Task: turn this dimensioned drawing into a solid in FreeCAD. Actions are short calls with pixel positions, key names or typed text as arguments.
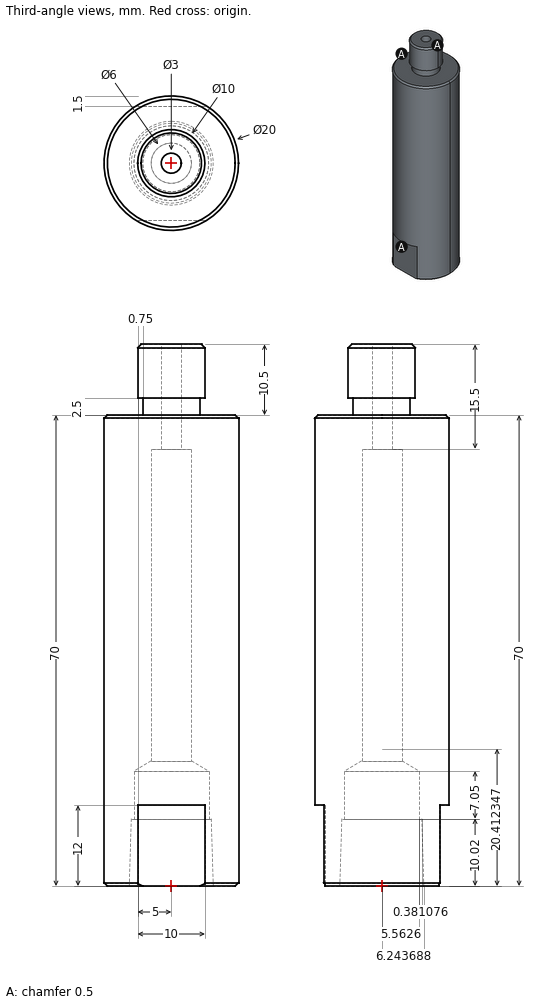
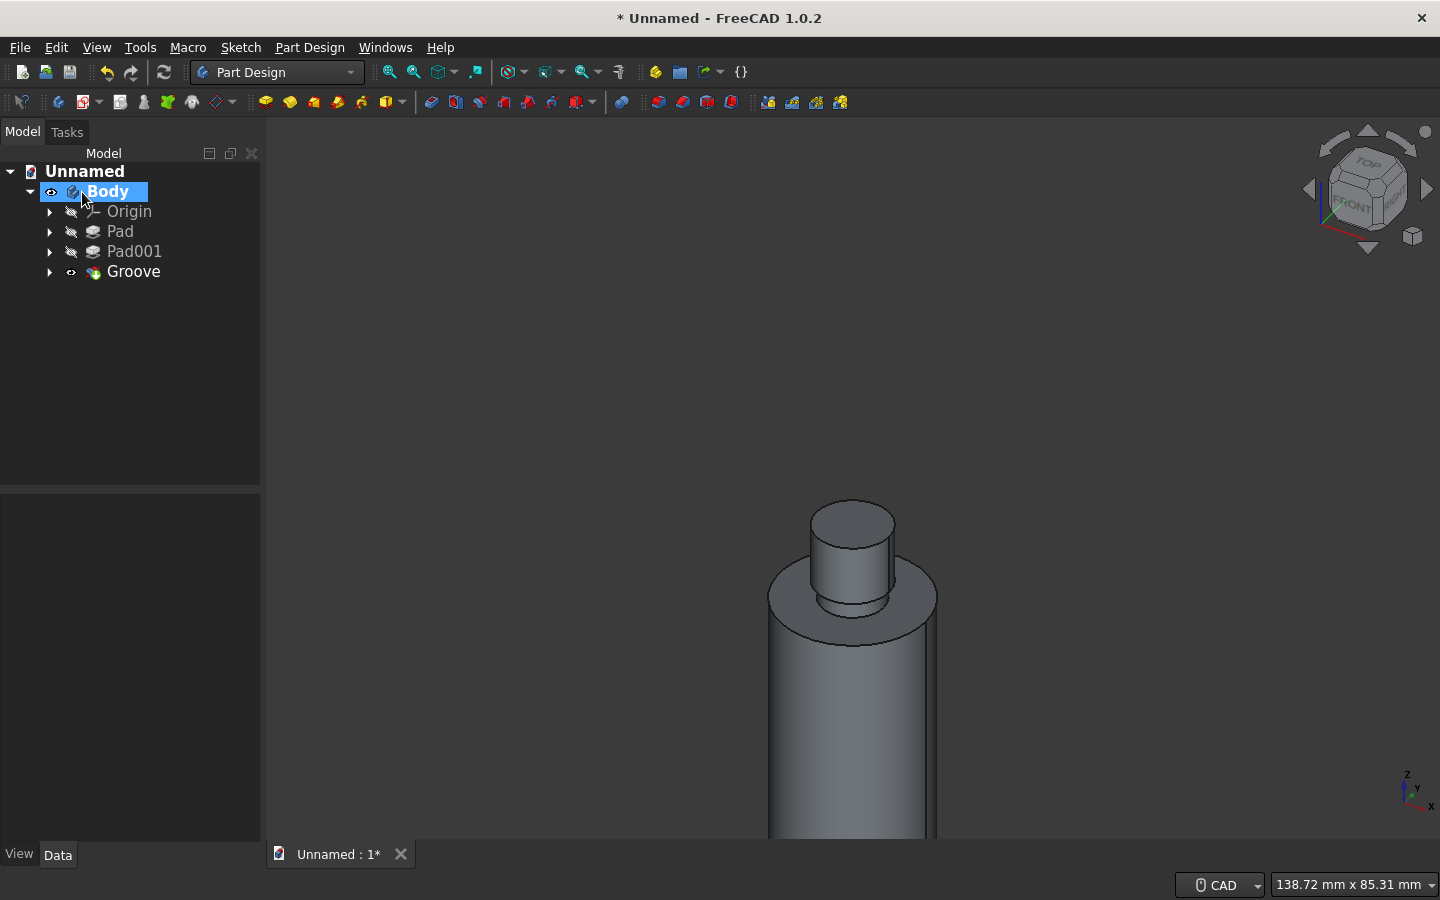
click(390, 72)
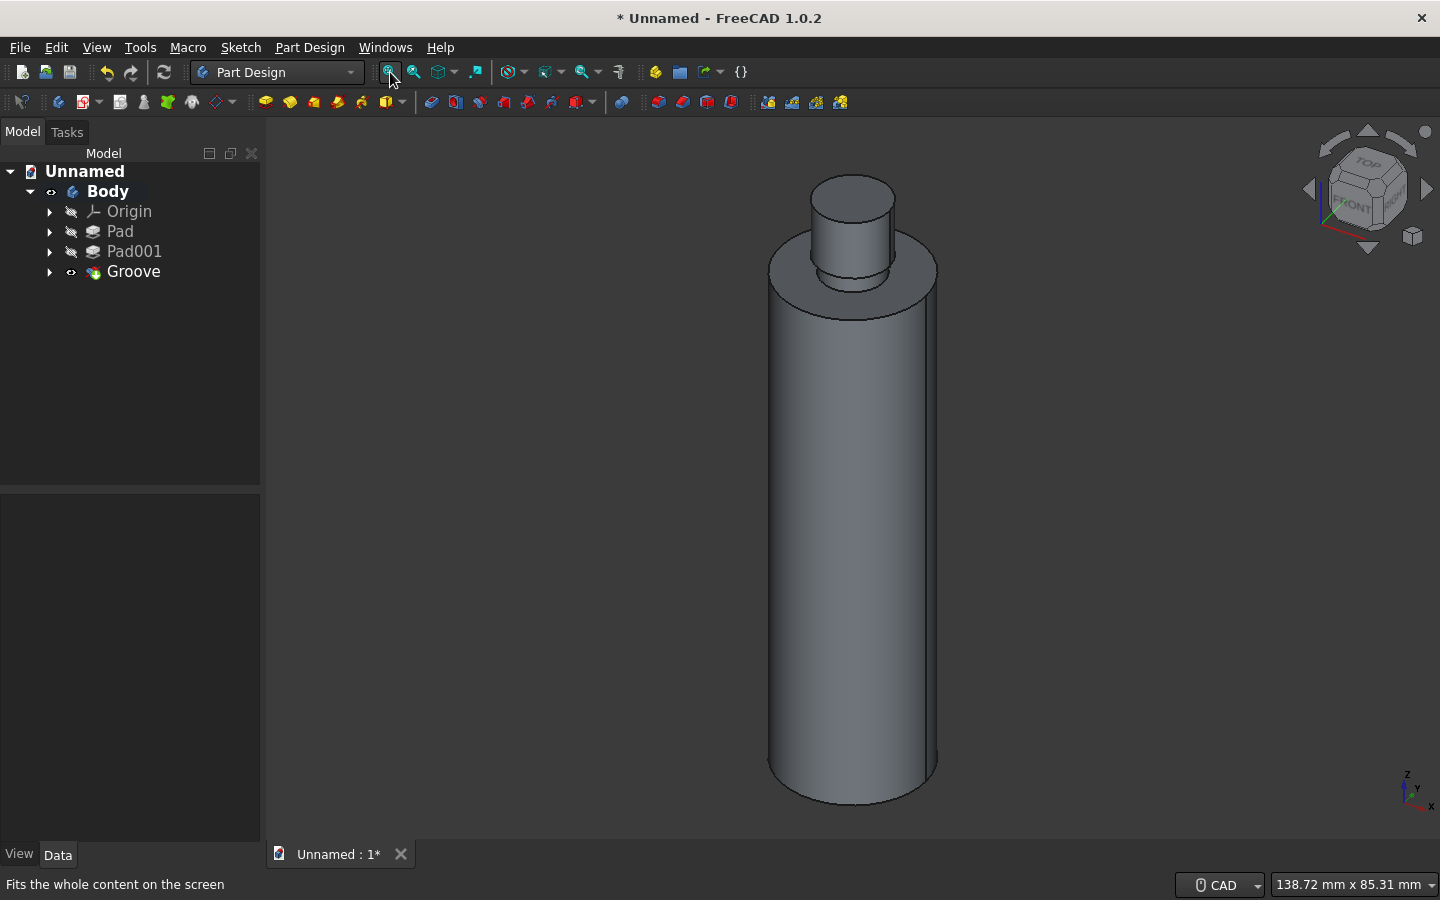
click(853, 198)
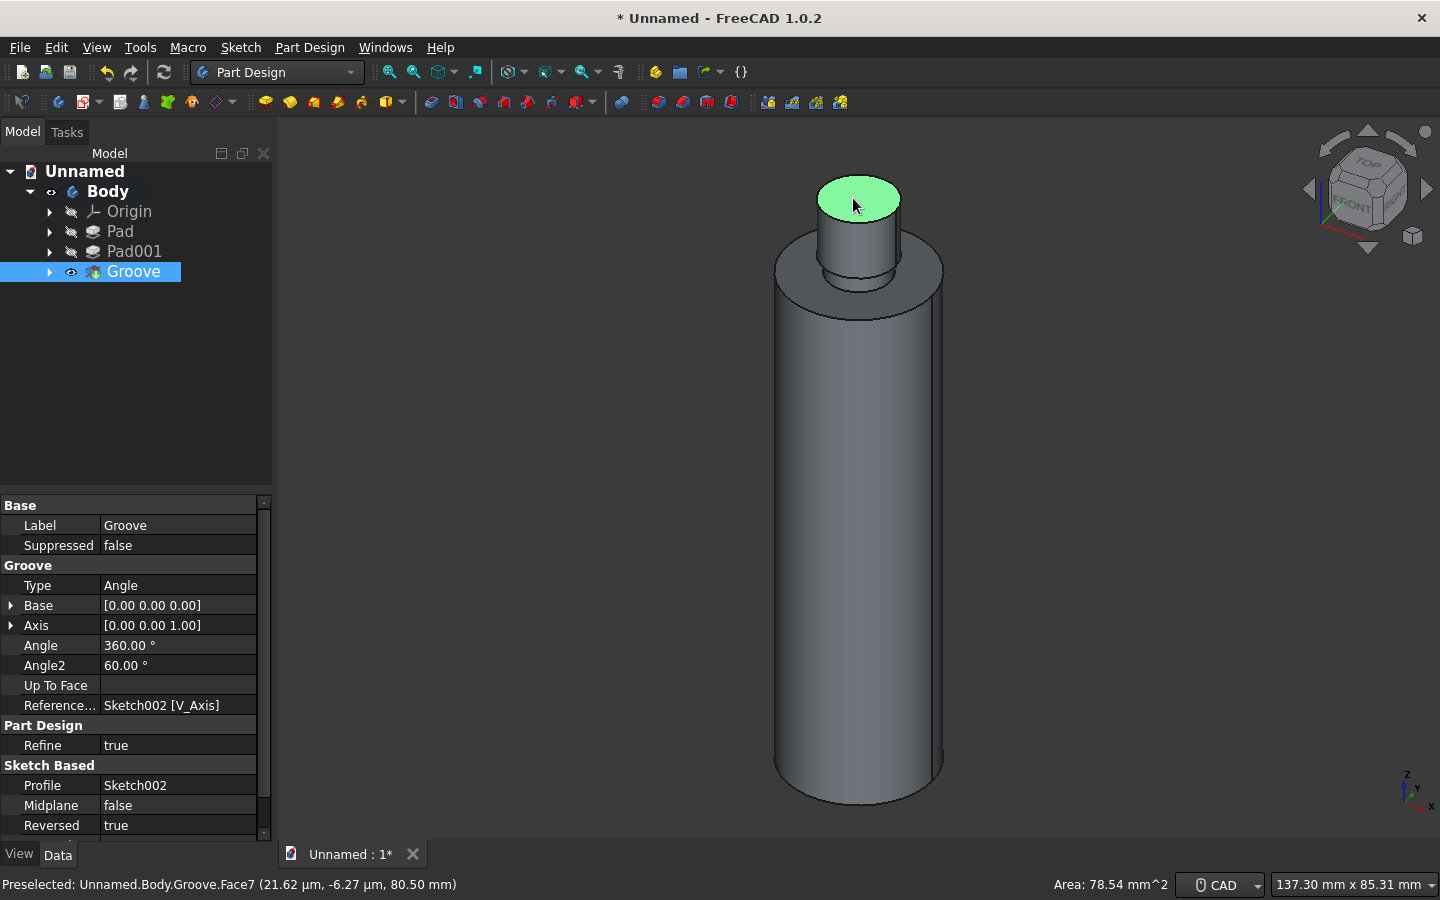
click(84, 102)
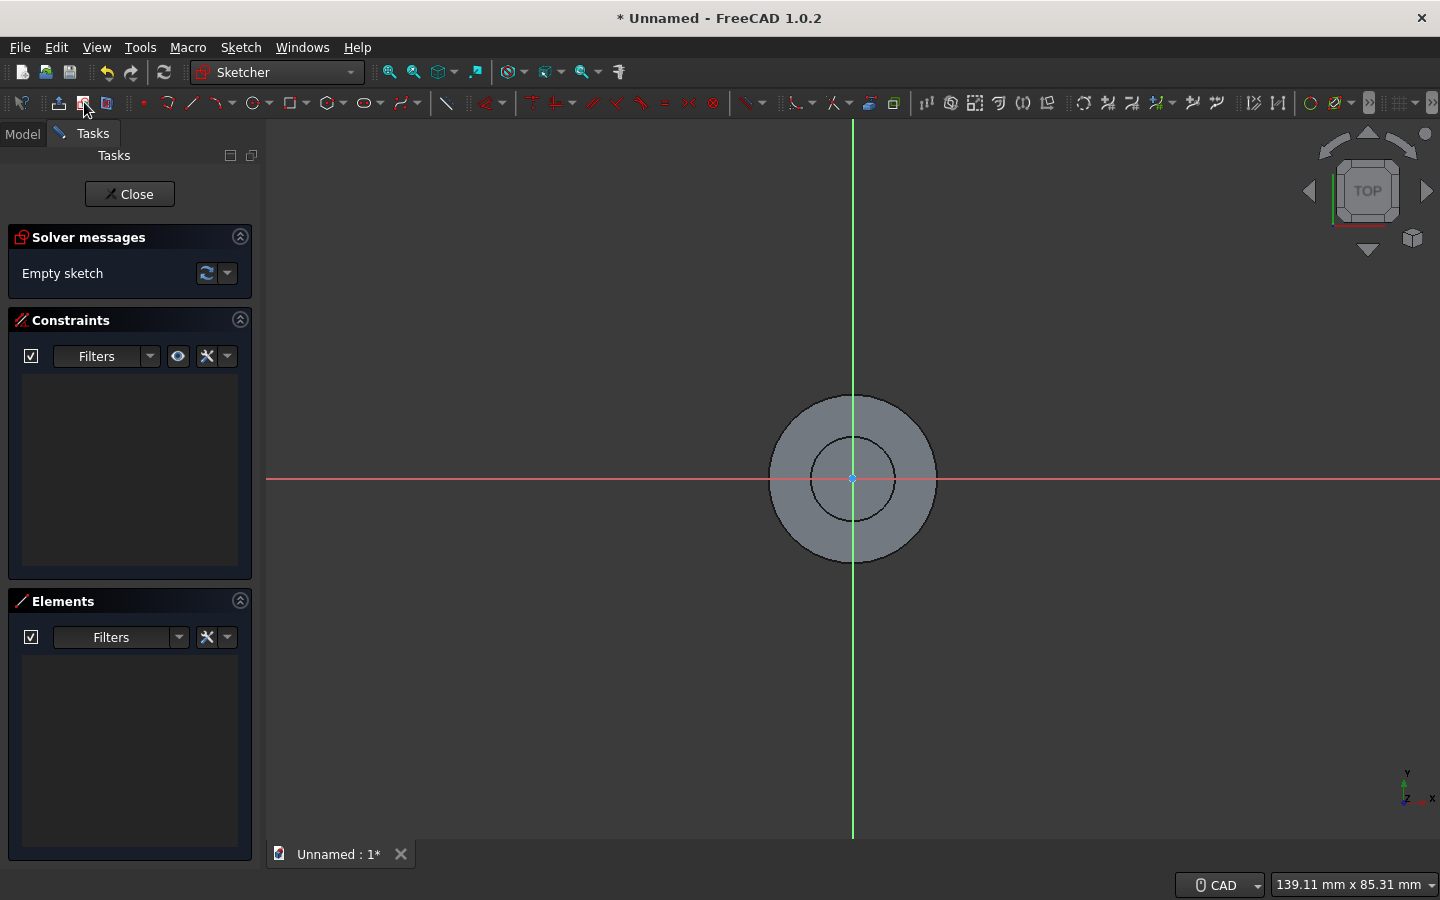
scroll(856, 479, up, 15)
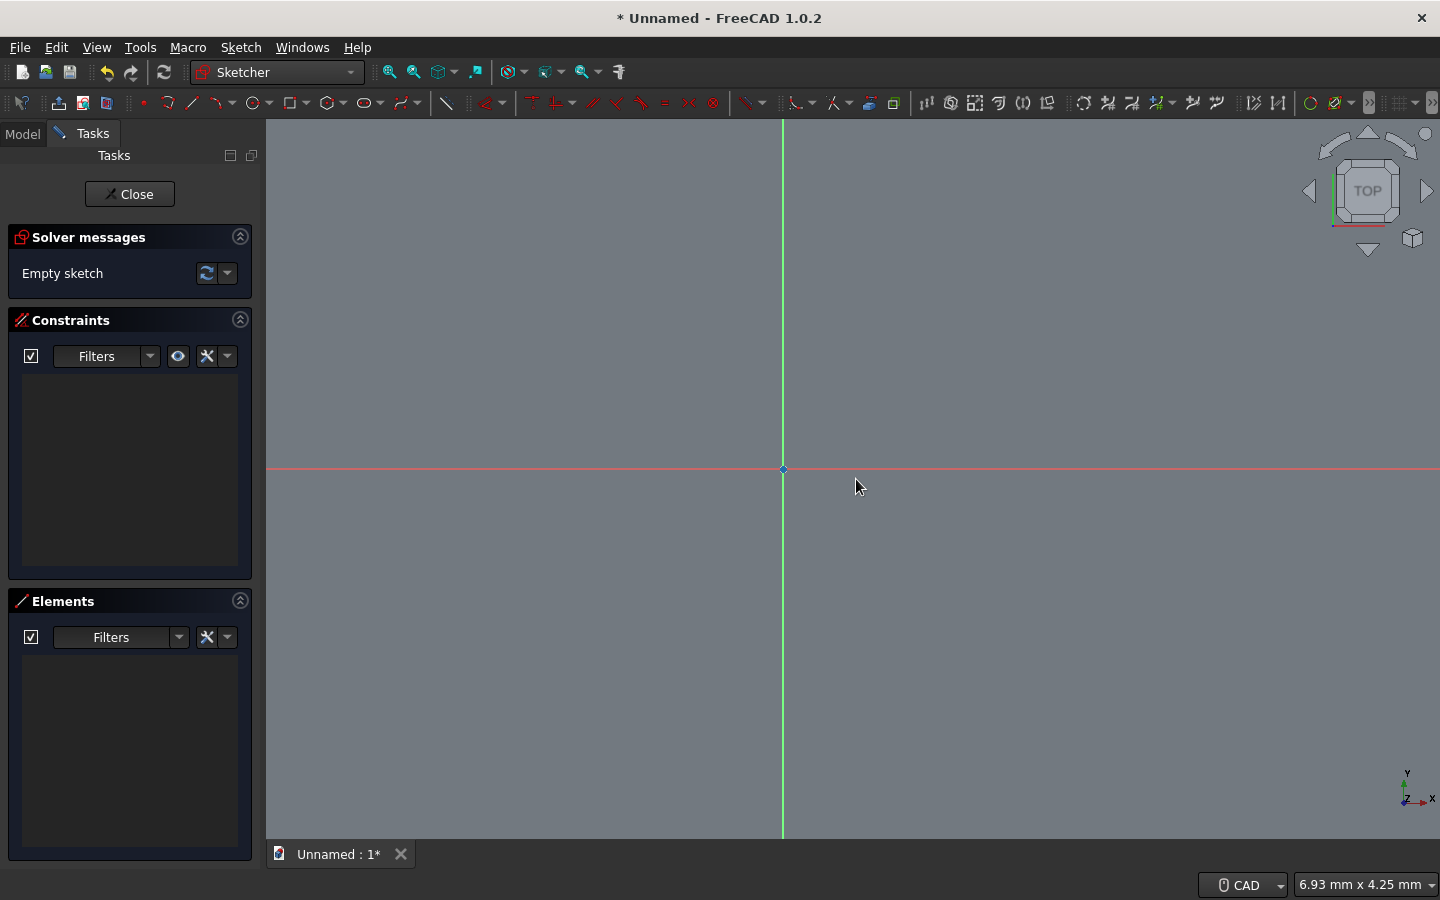
key(g)
key(c)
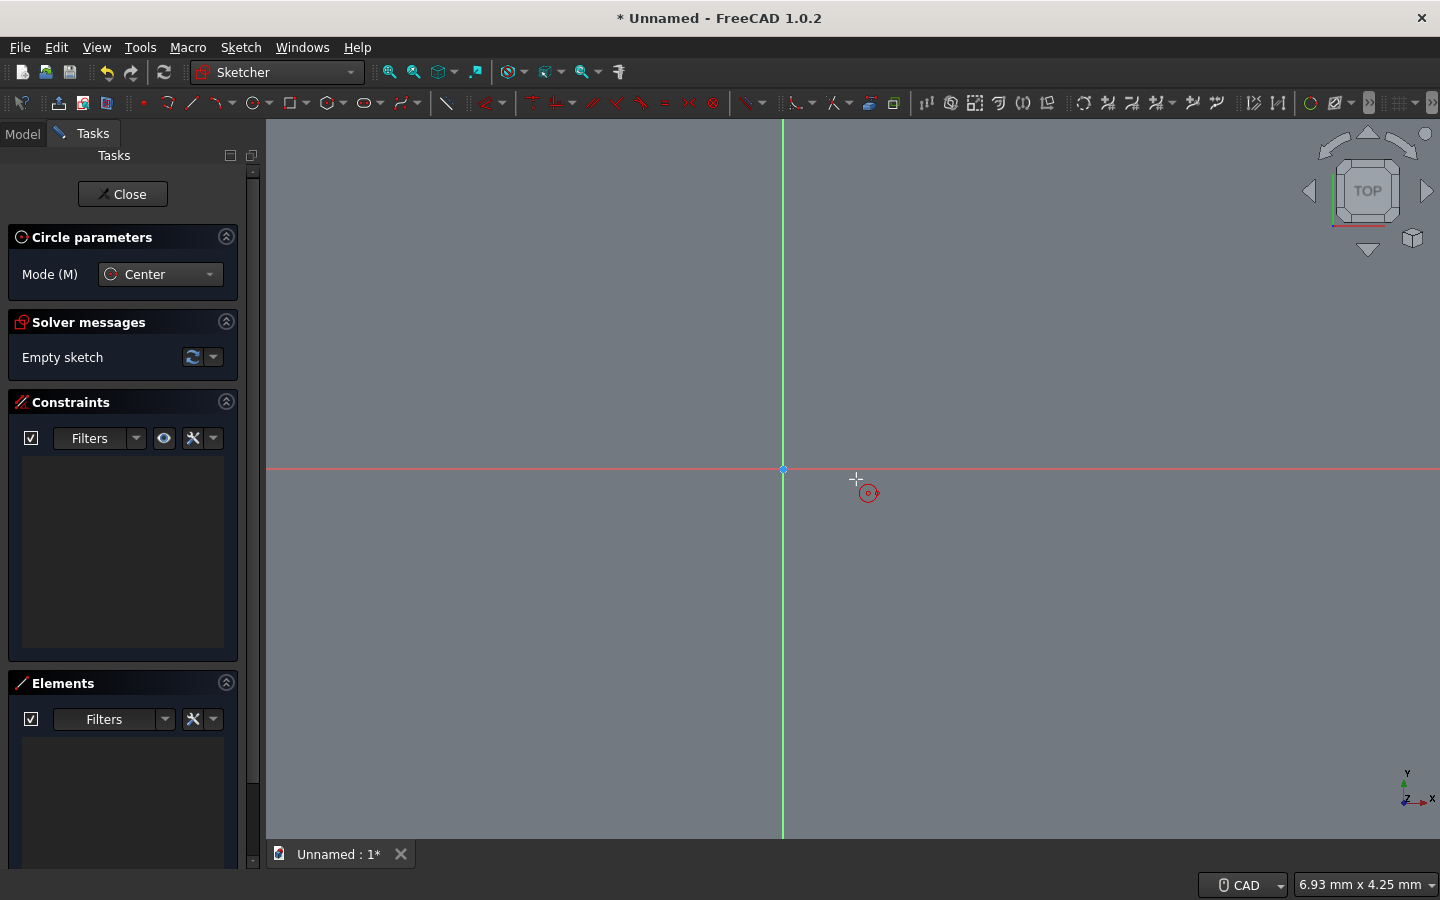
click(783, 469)
move(963, 290)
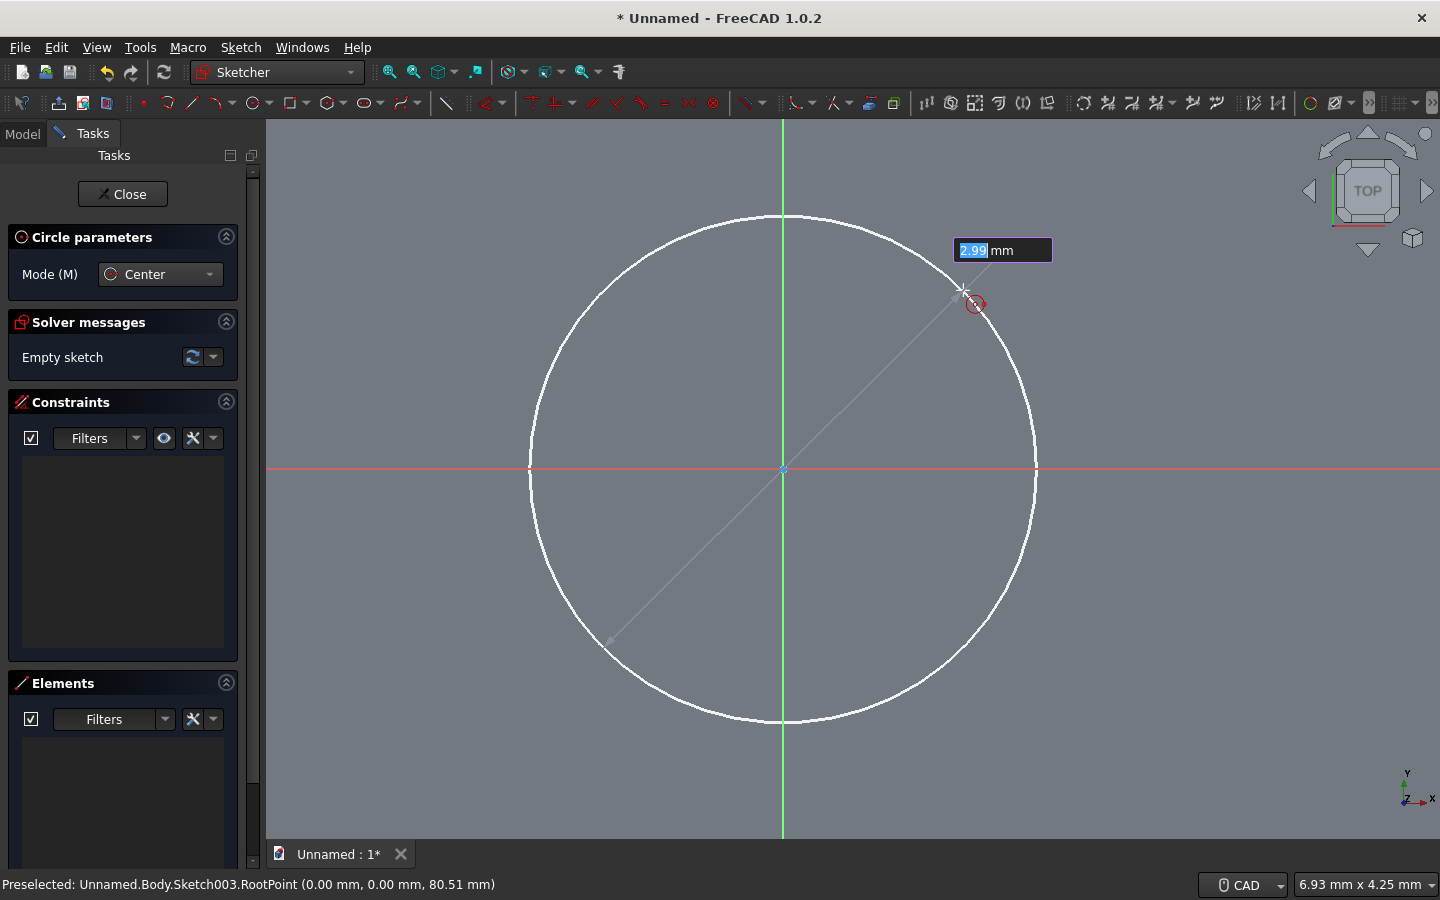
text(3)
key(Return)
key(Escape)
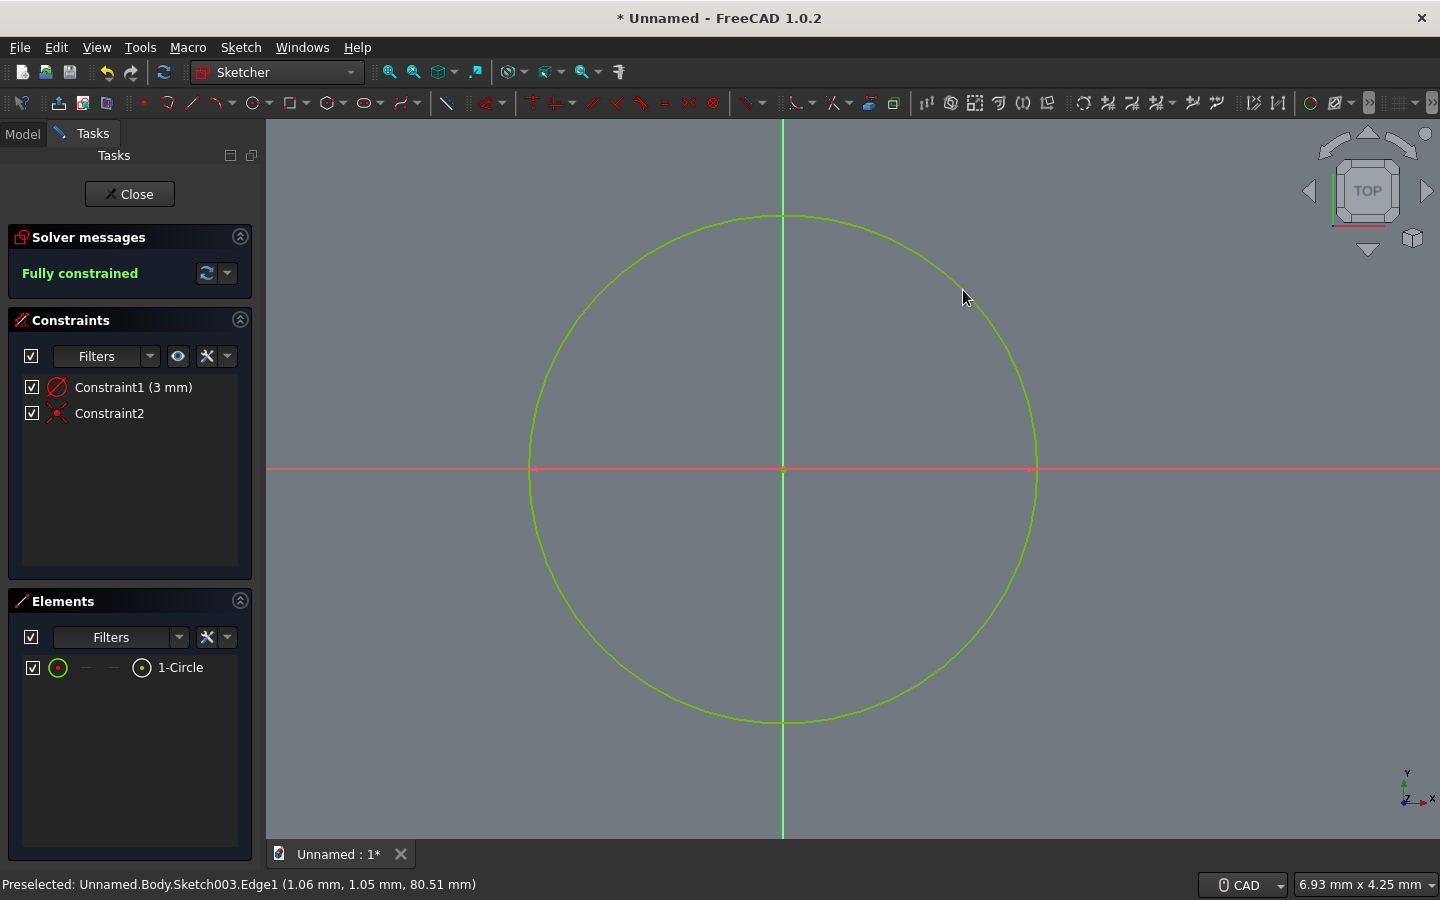
click(130, 194)